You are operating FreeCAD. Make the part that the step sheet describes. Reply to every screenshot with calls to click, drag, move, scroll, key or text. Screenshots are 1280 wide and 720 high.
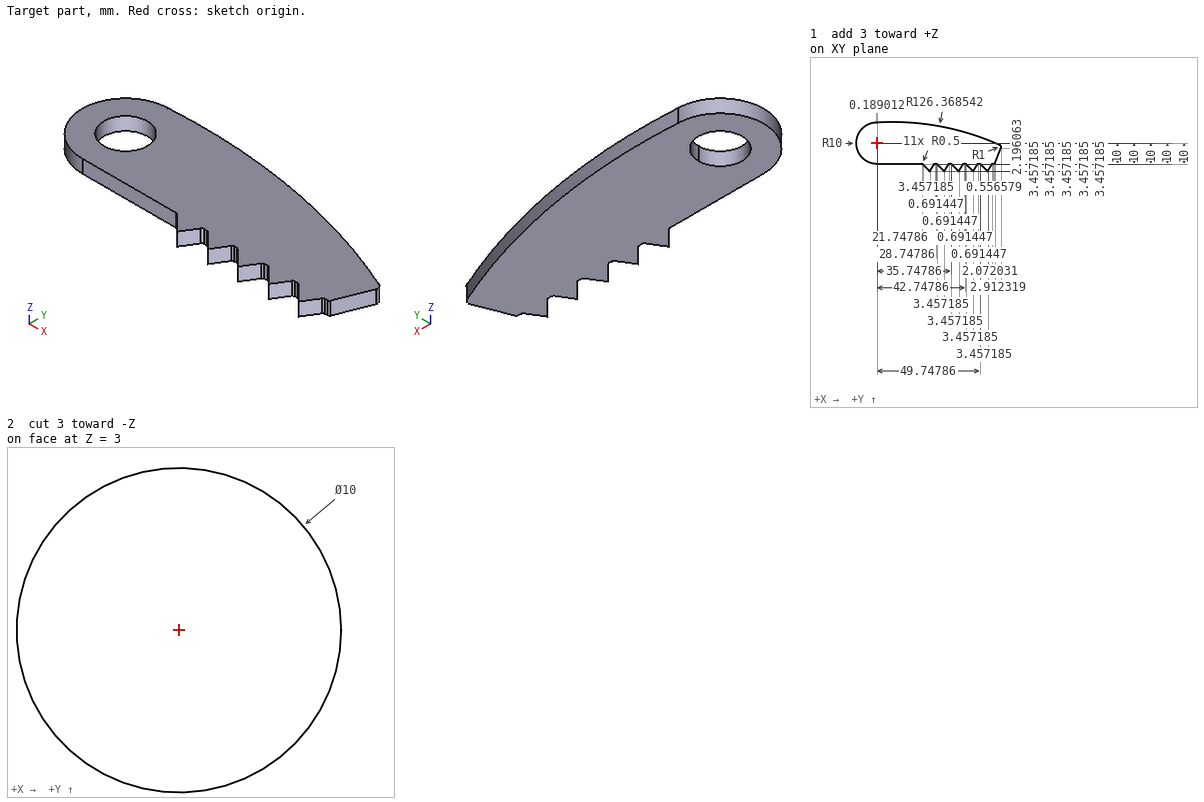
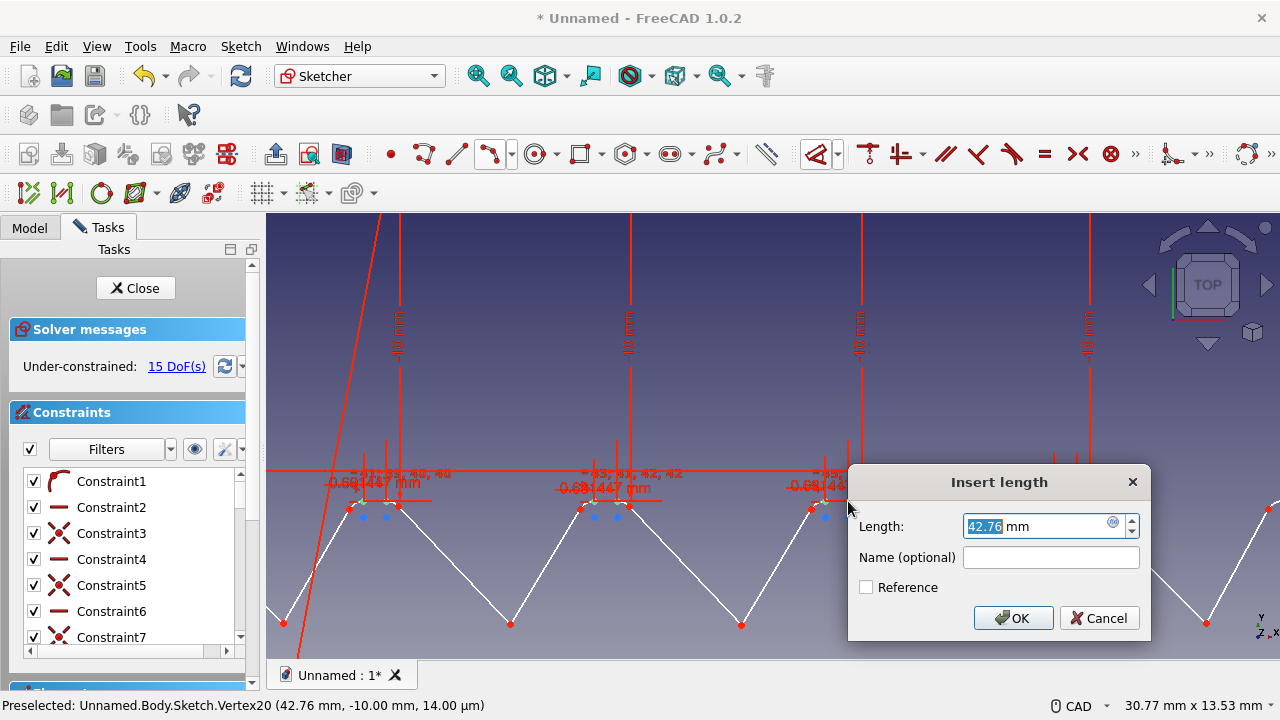
text(42.74786)
key(Return)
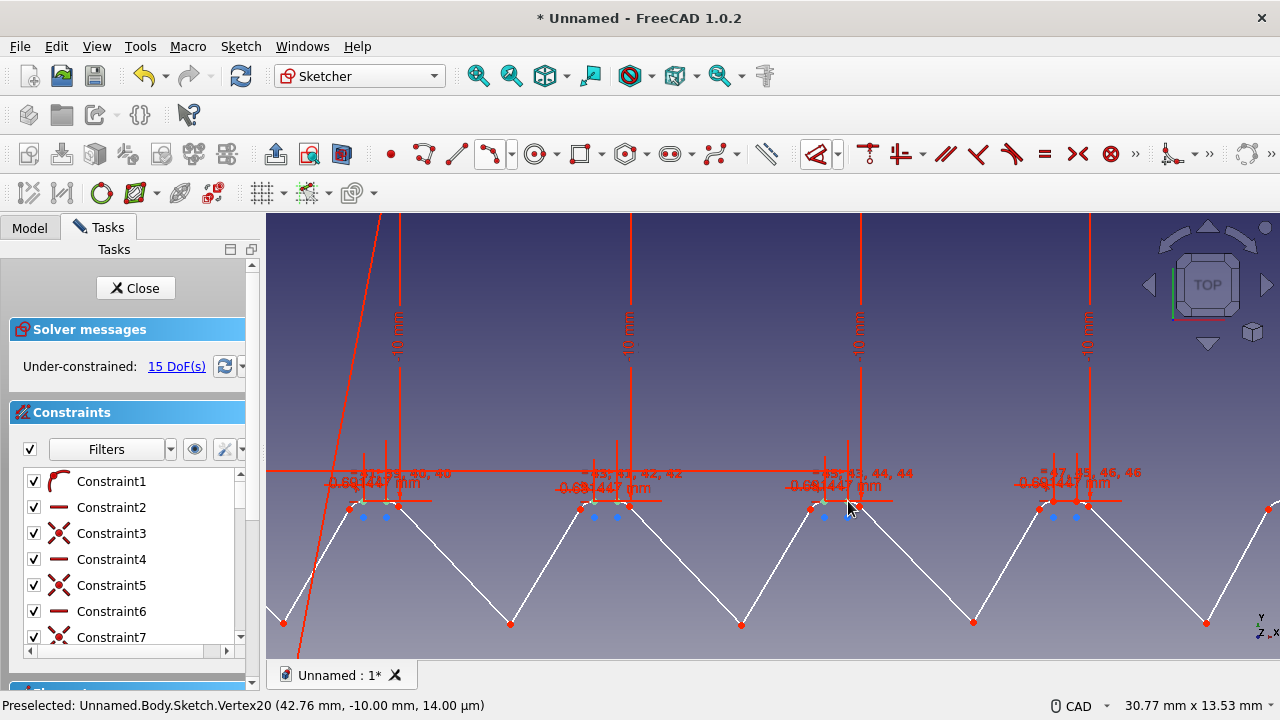
click(1077, 501)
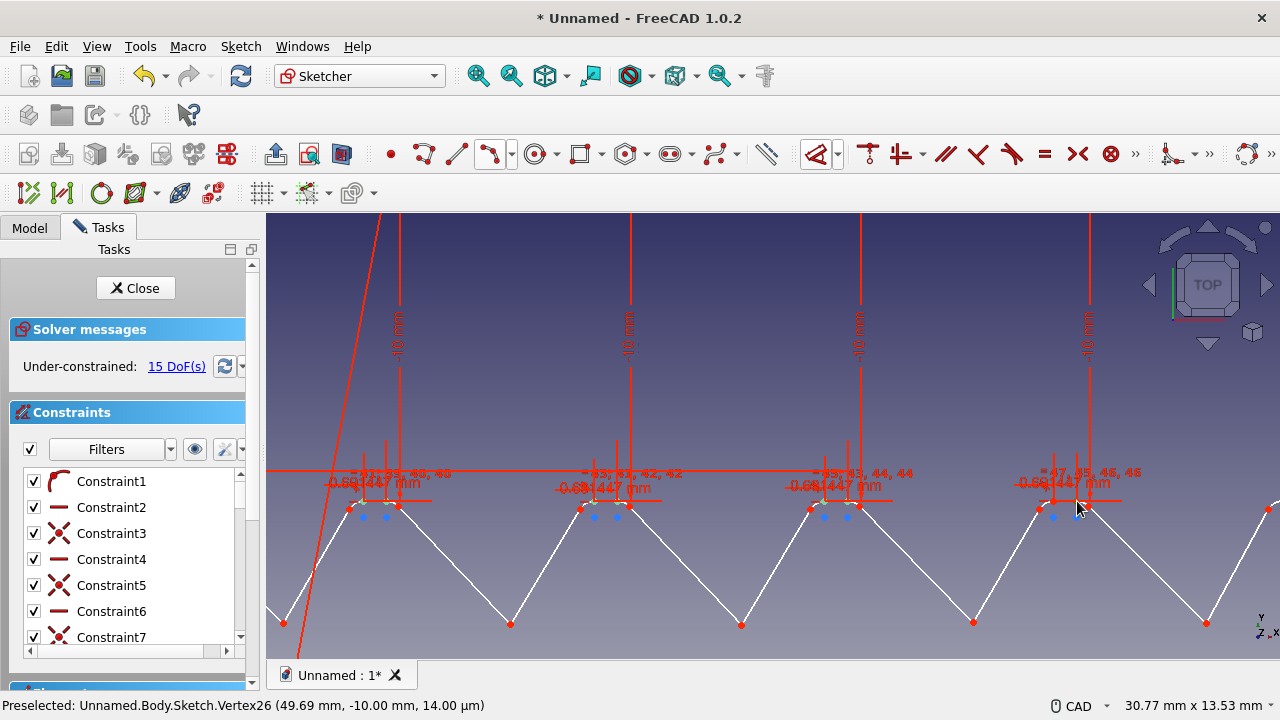
key(l)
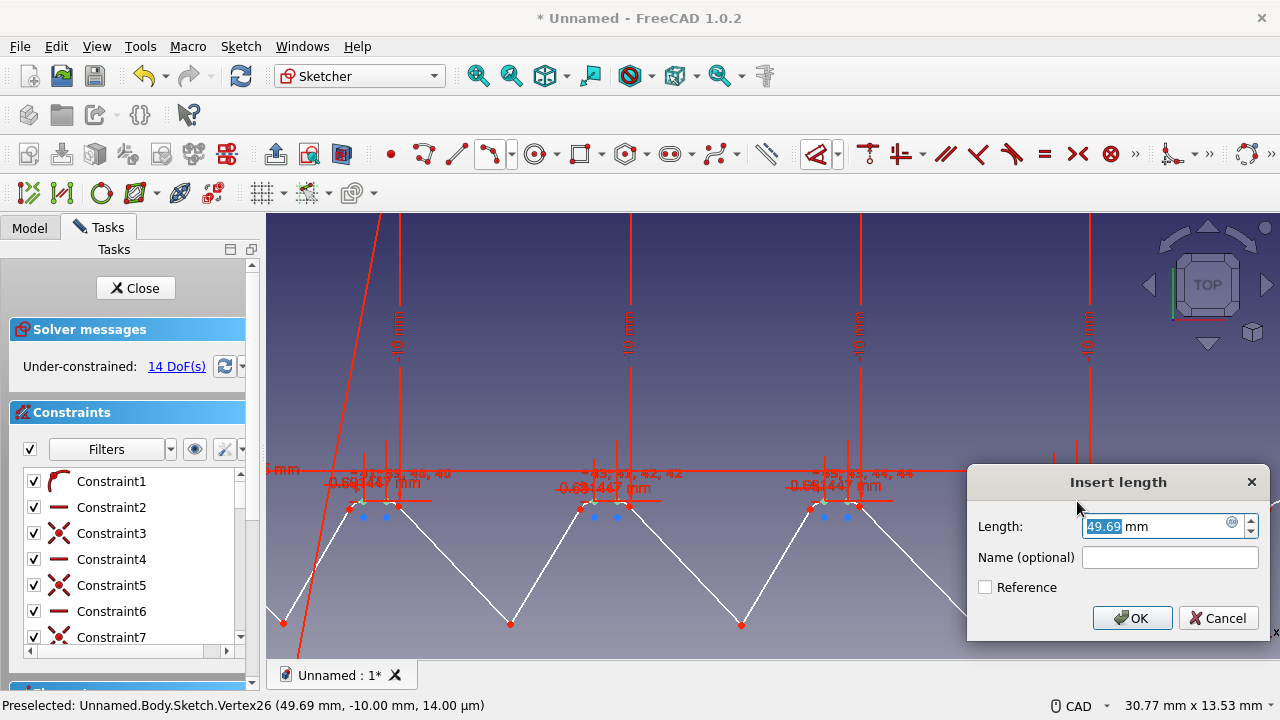
text(49.74786)
key(Return)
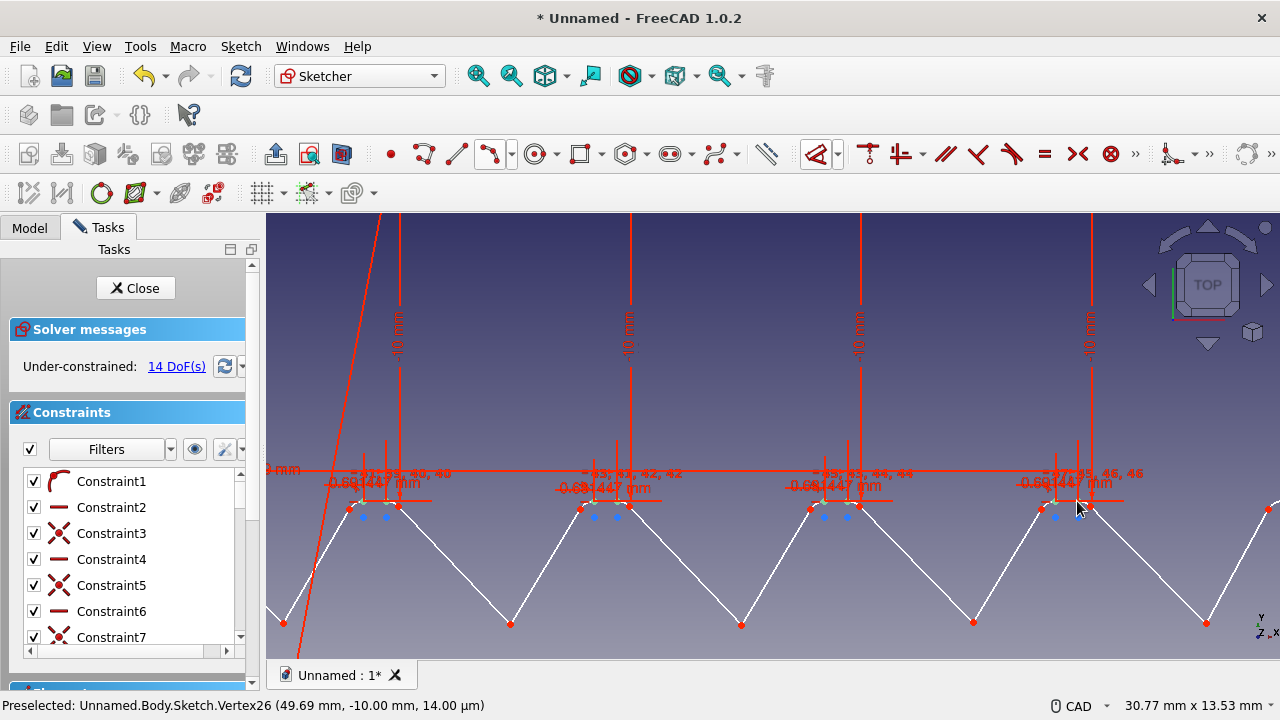
scroll(849, 503, down, 7)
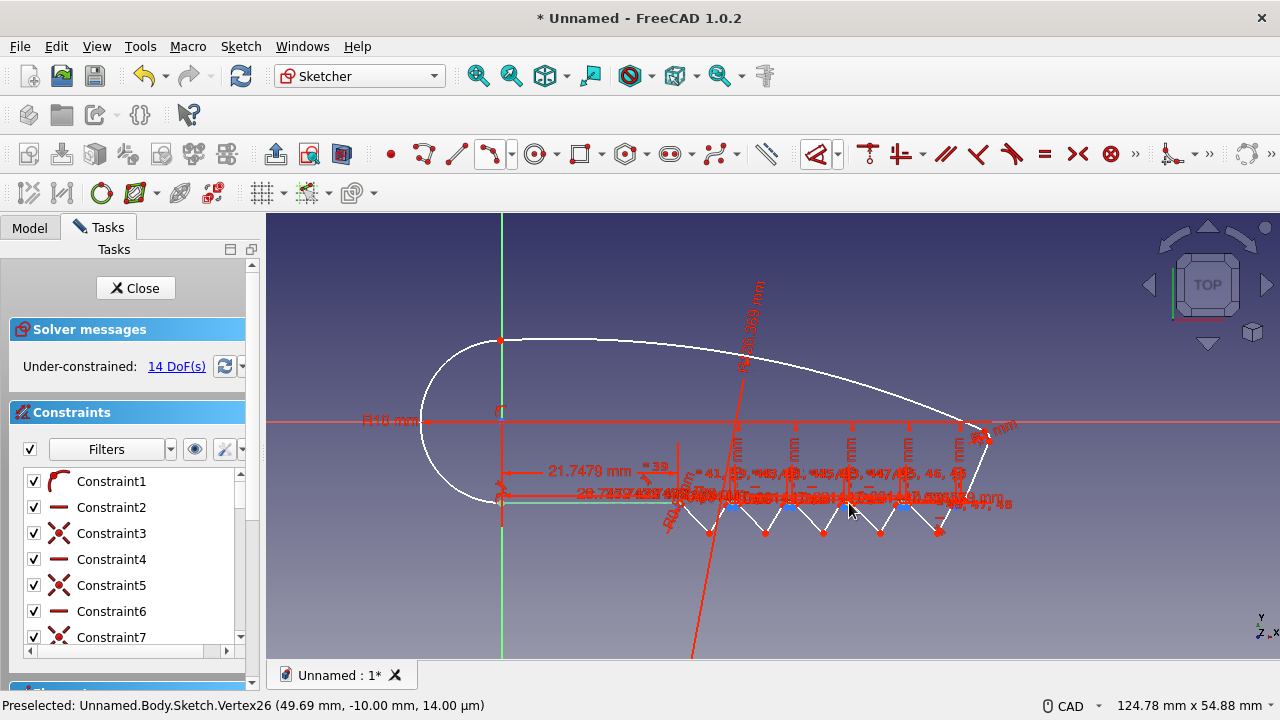
scroll(989, 442, up, 4)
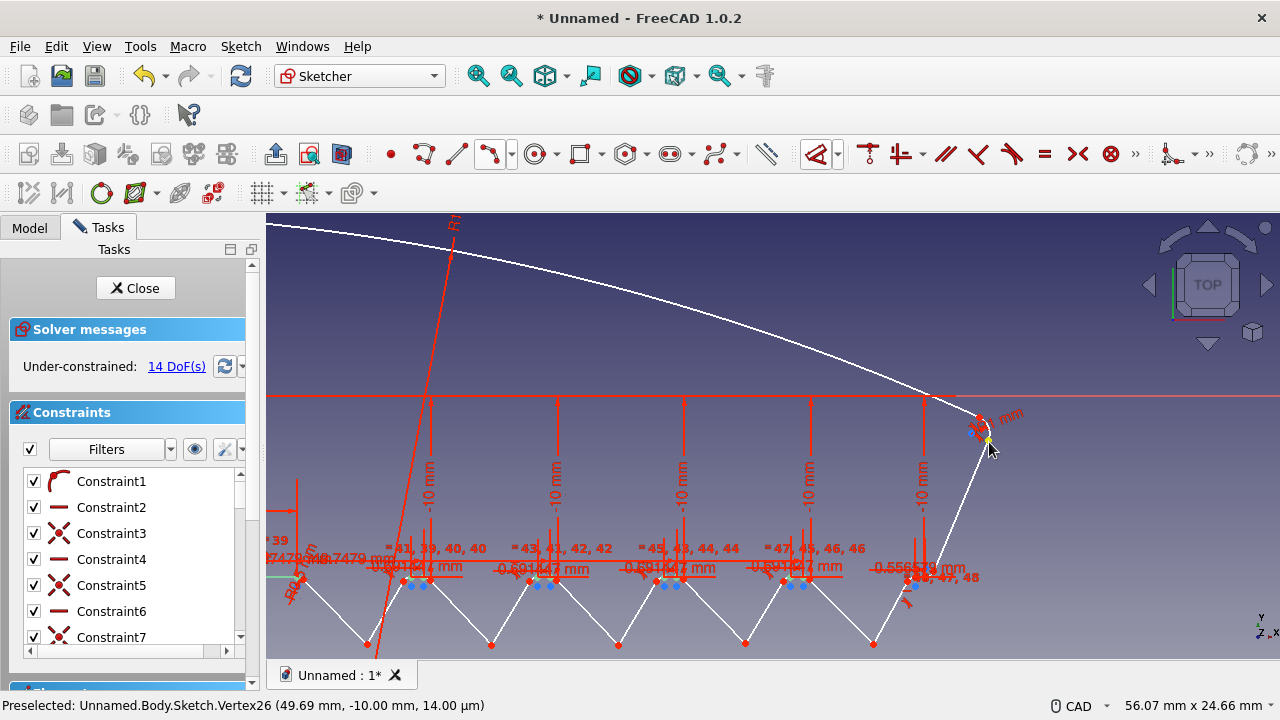
click(988, 441)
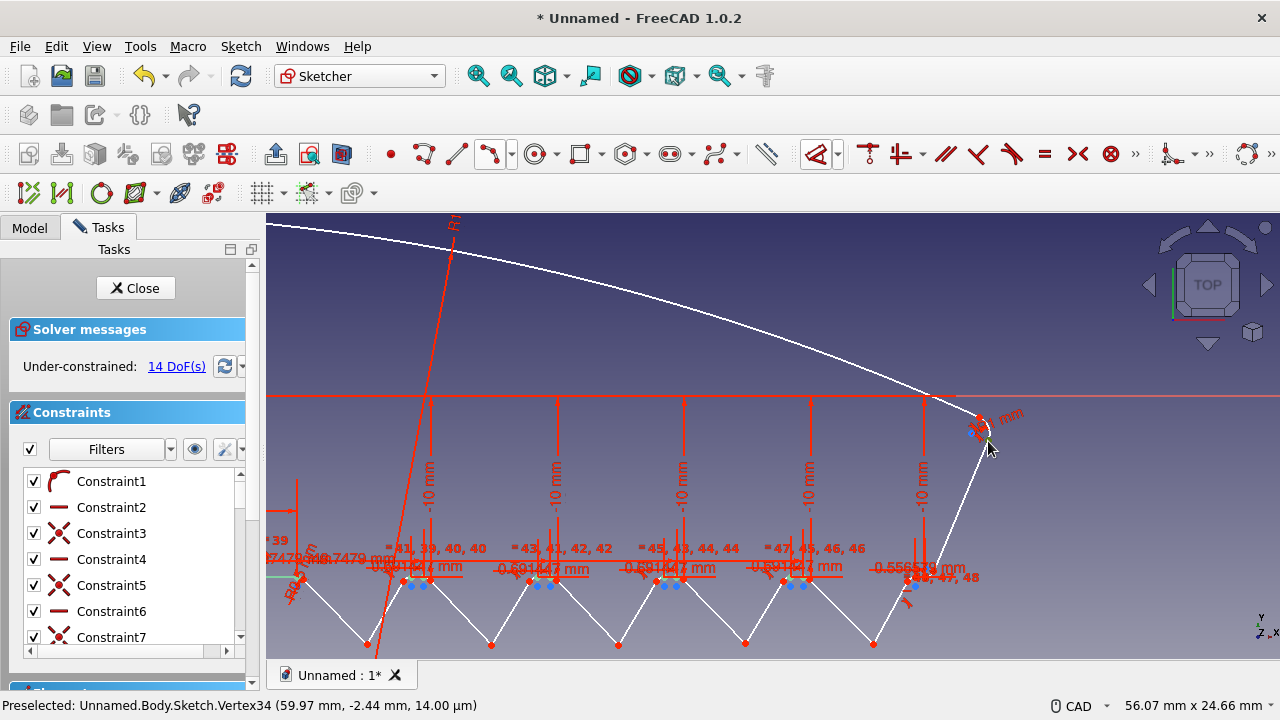
click(838, 154)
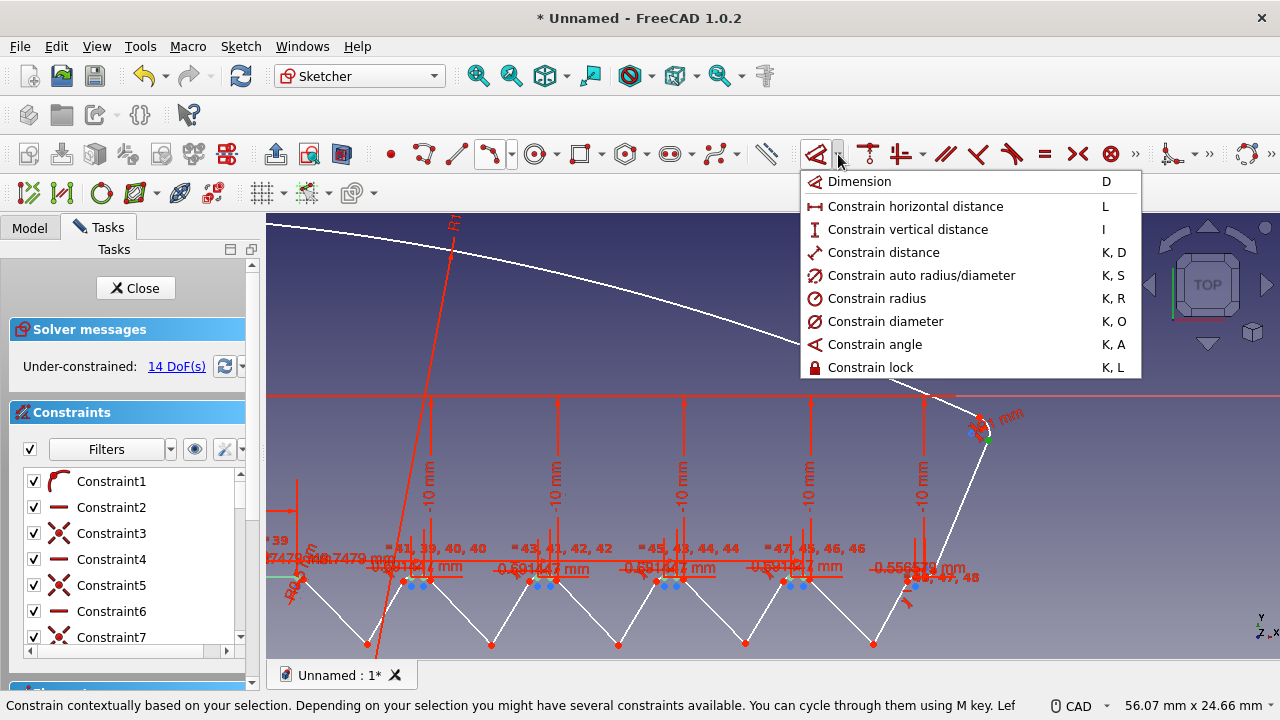
click(971, 230)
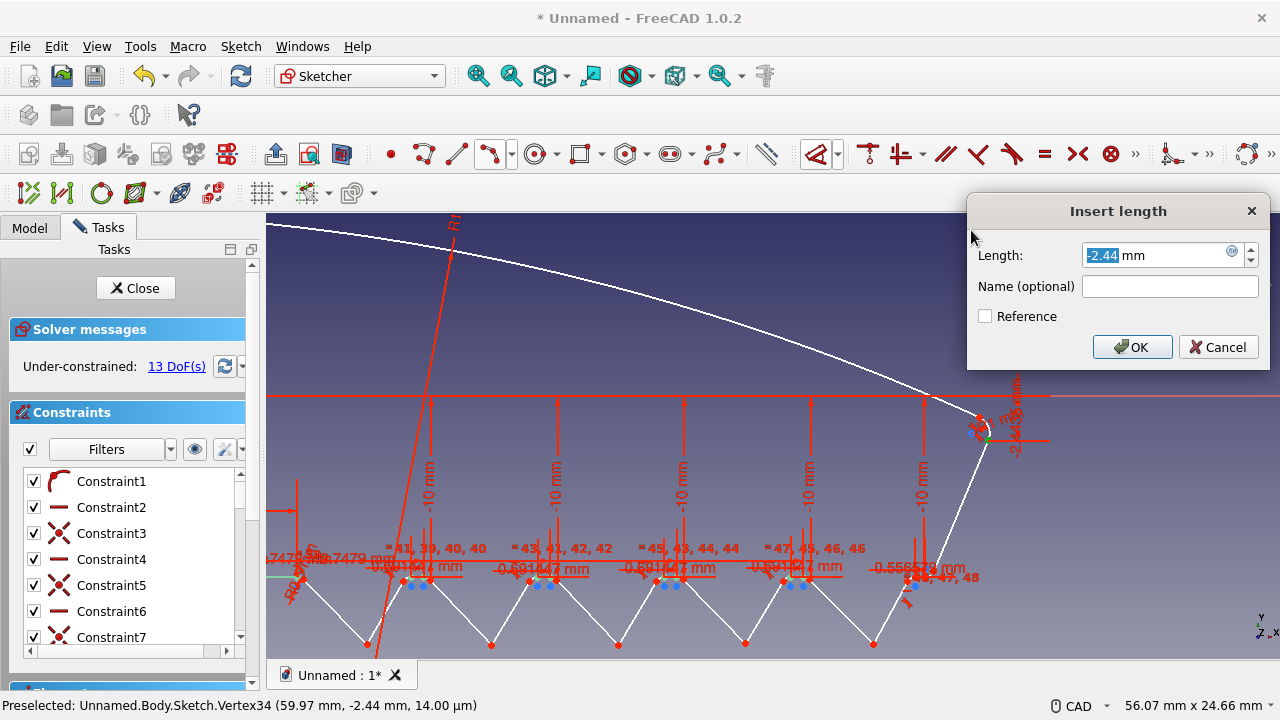
text(-2.196063)
key(Return)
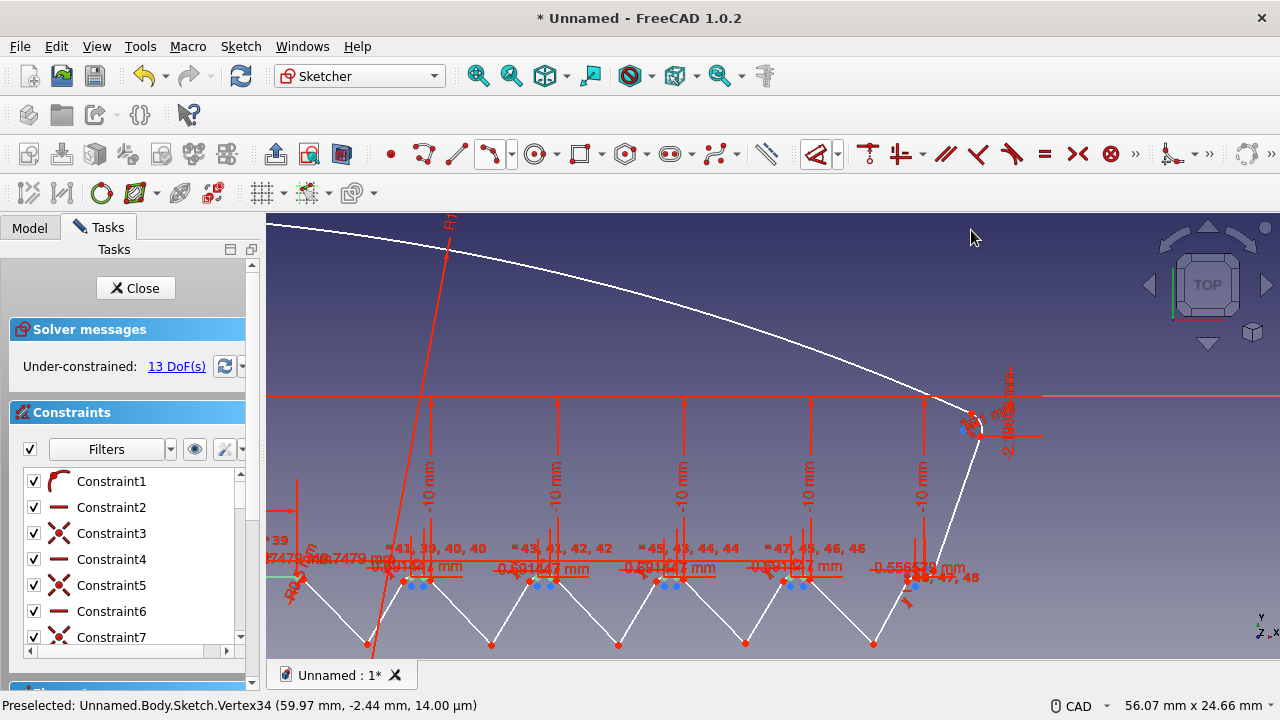
scroll(989, 442, down, 4)